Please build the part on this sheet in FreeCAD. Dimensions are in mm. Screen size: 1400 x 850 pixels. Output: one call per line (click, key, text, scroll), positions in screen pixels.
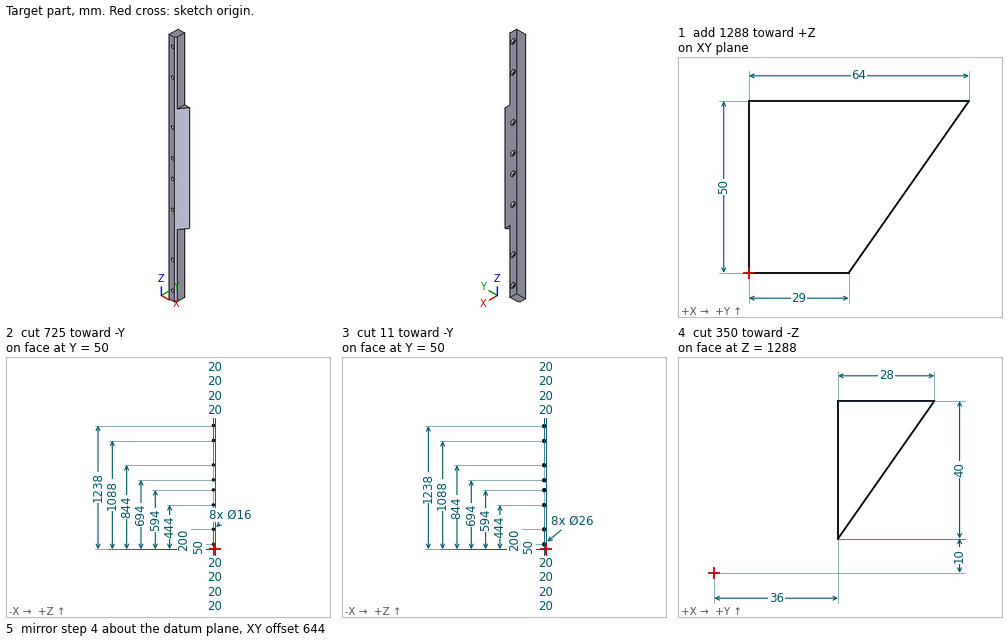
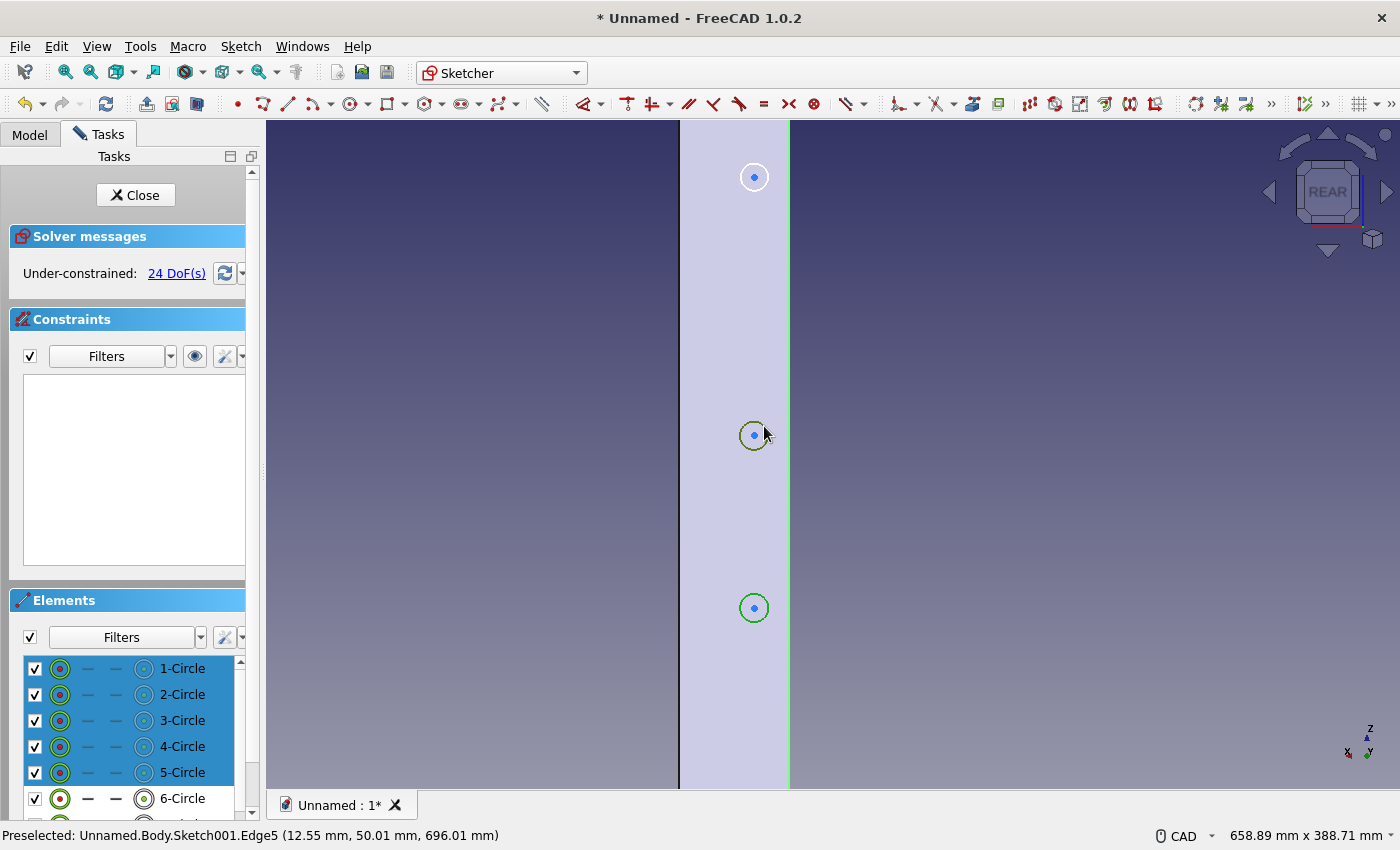
click(764, 167)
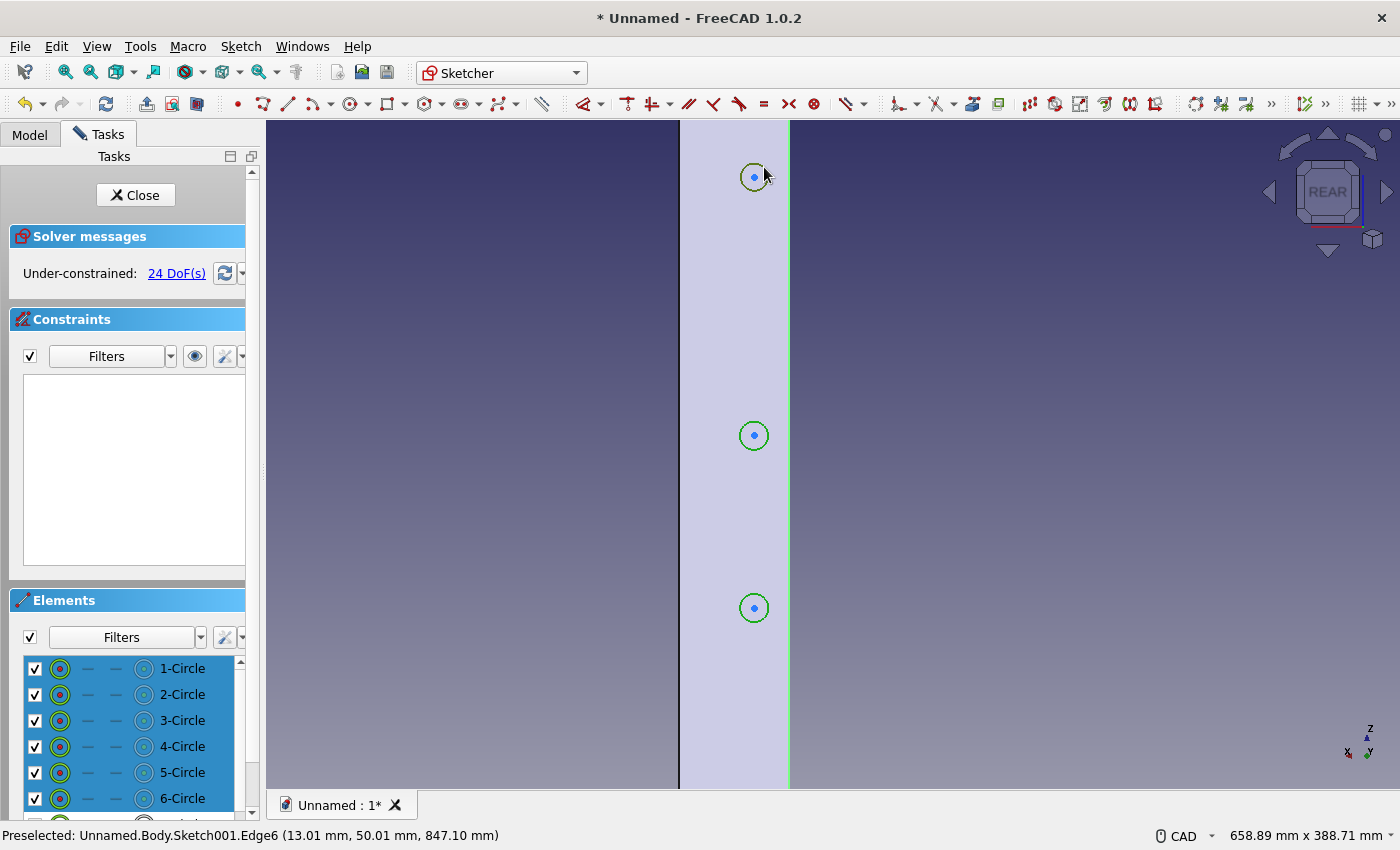
scroll(764, 429, down, 8)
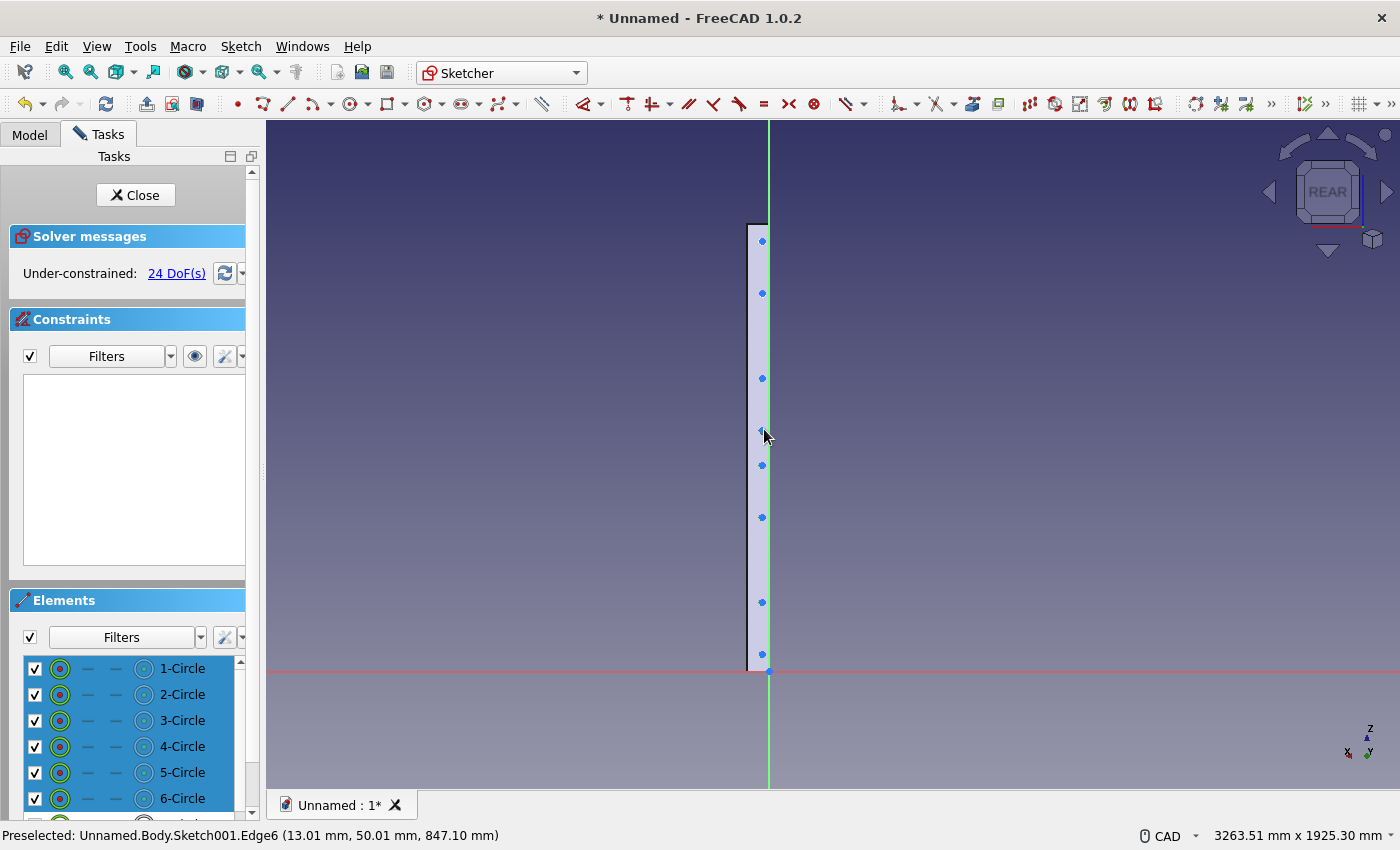
scroll(765, 292, up, 8)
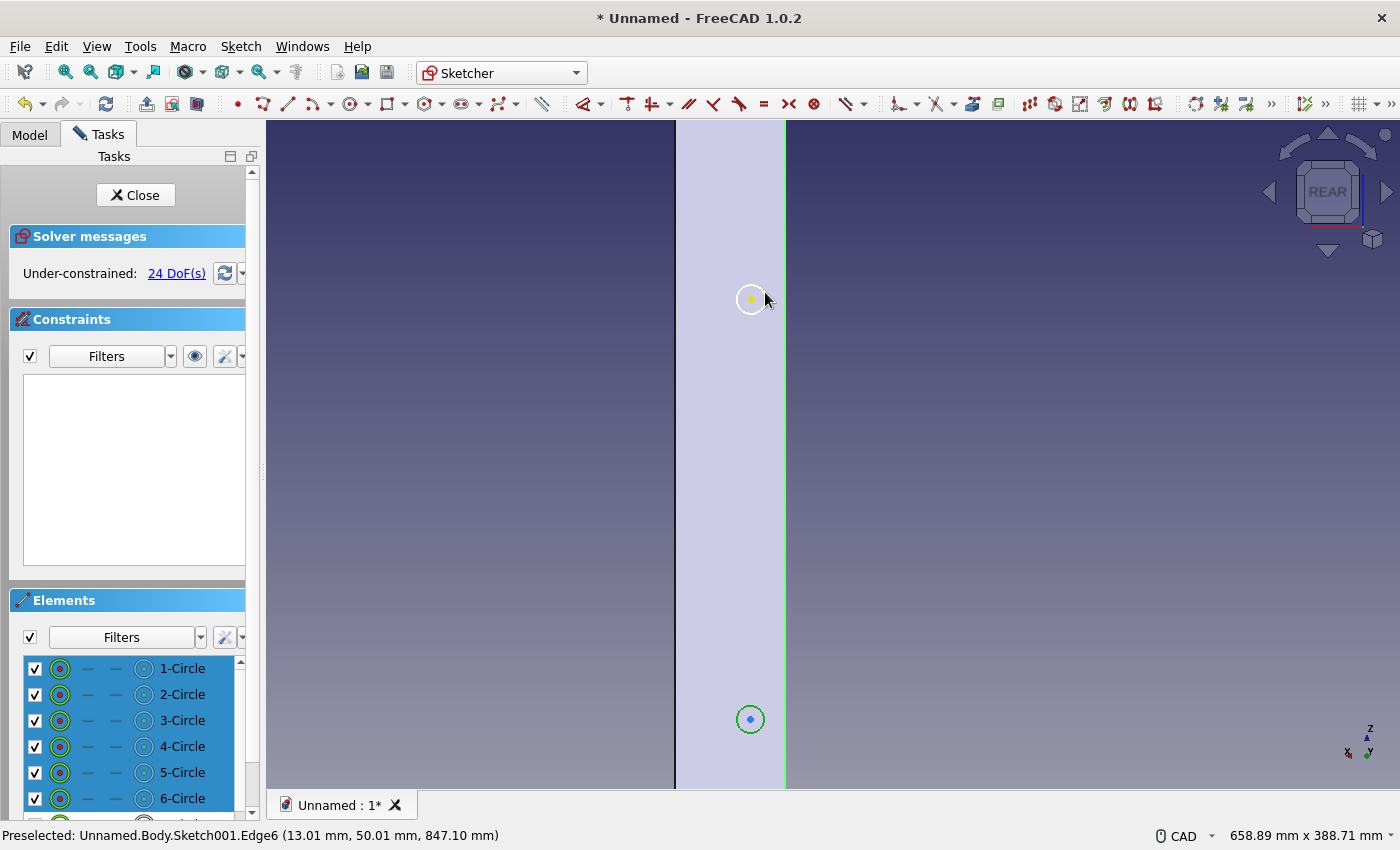
click(761, 289)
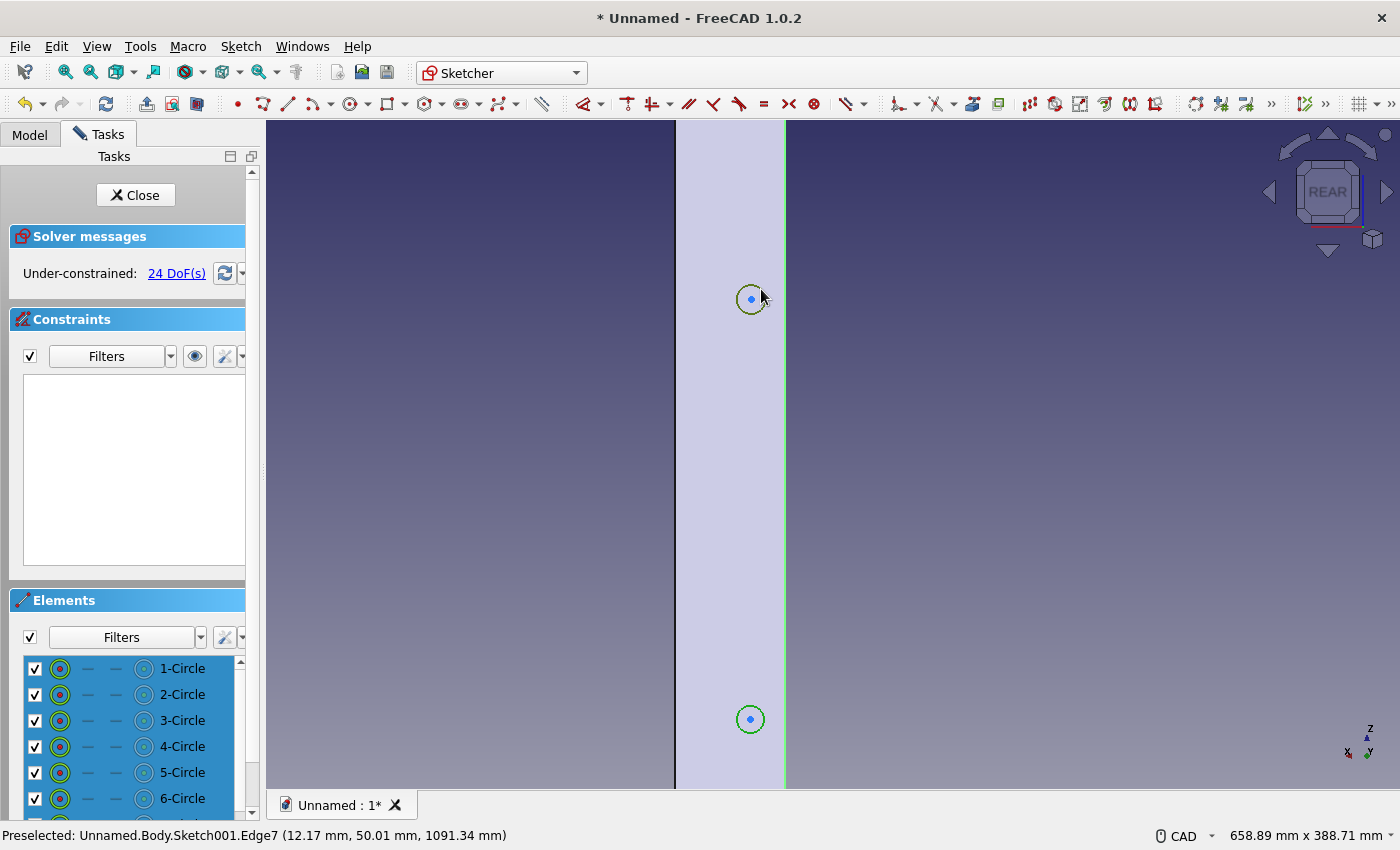
scroll(765, 292, down, 8)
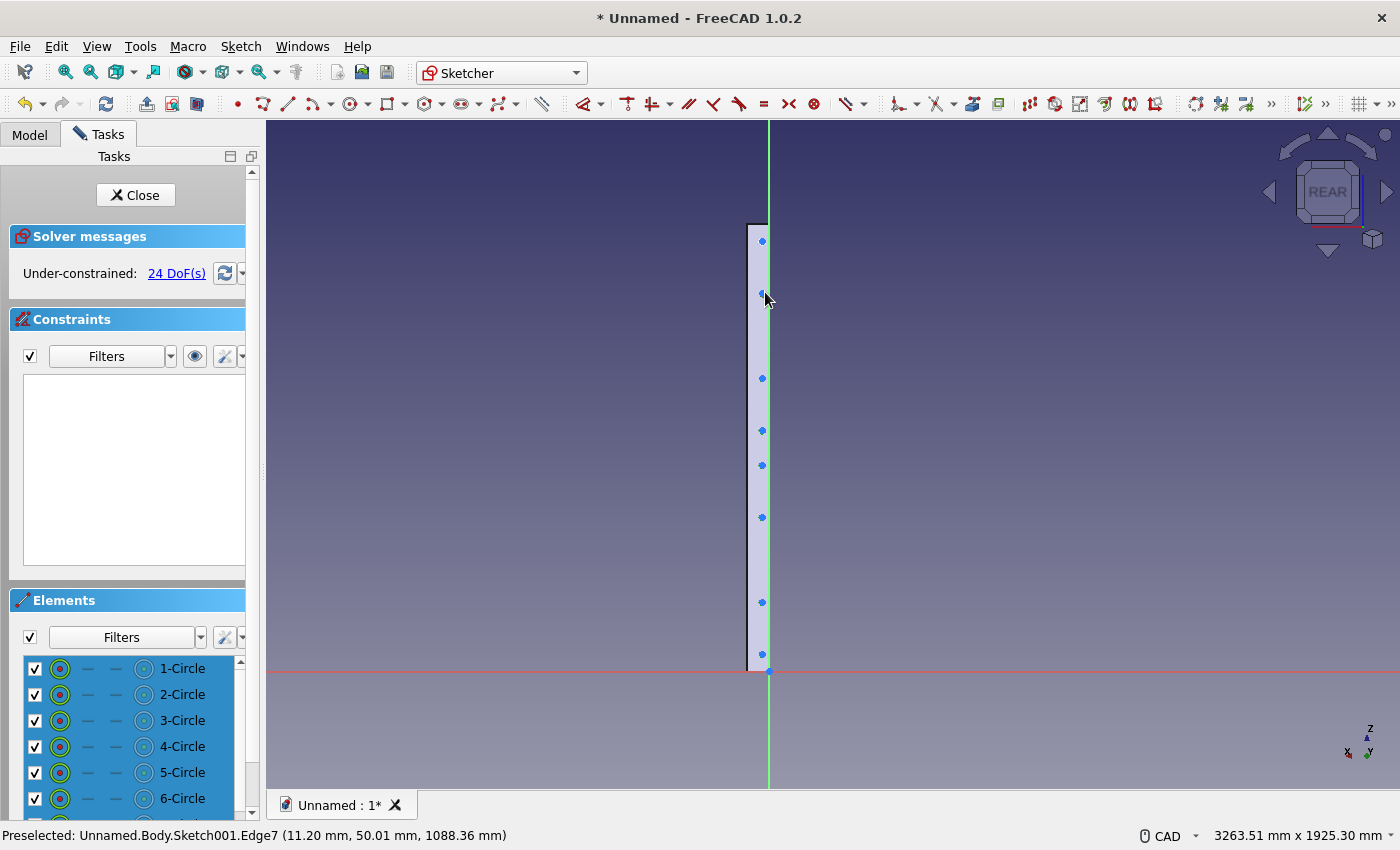
scroll(764, 240, up, 8)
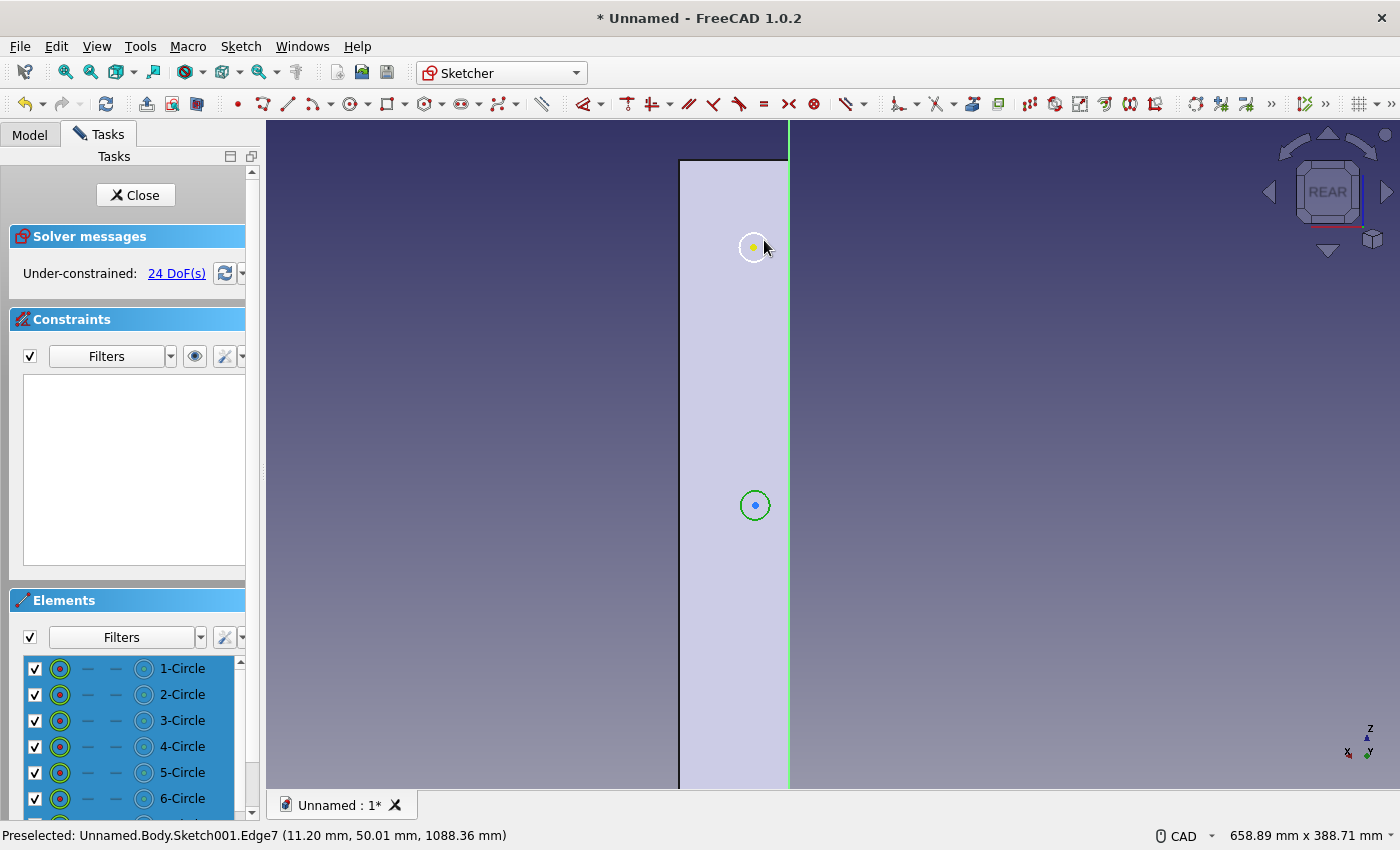
click(764, 237)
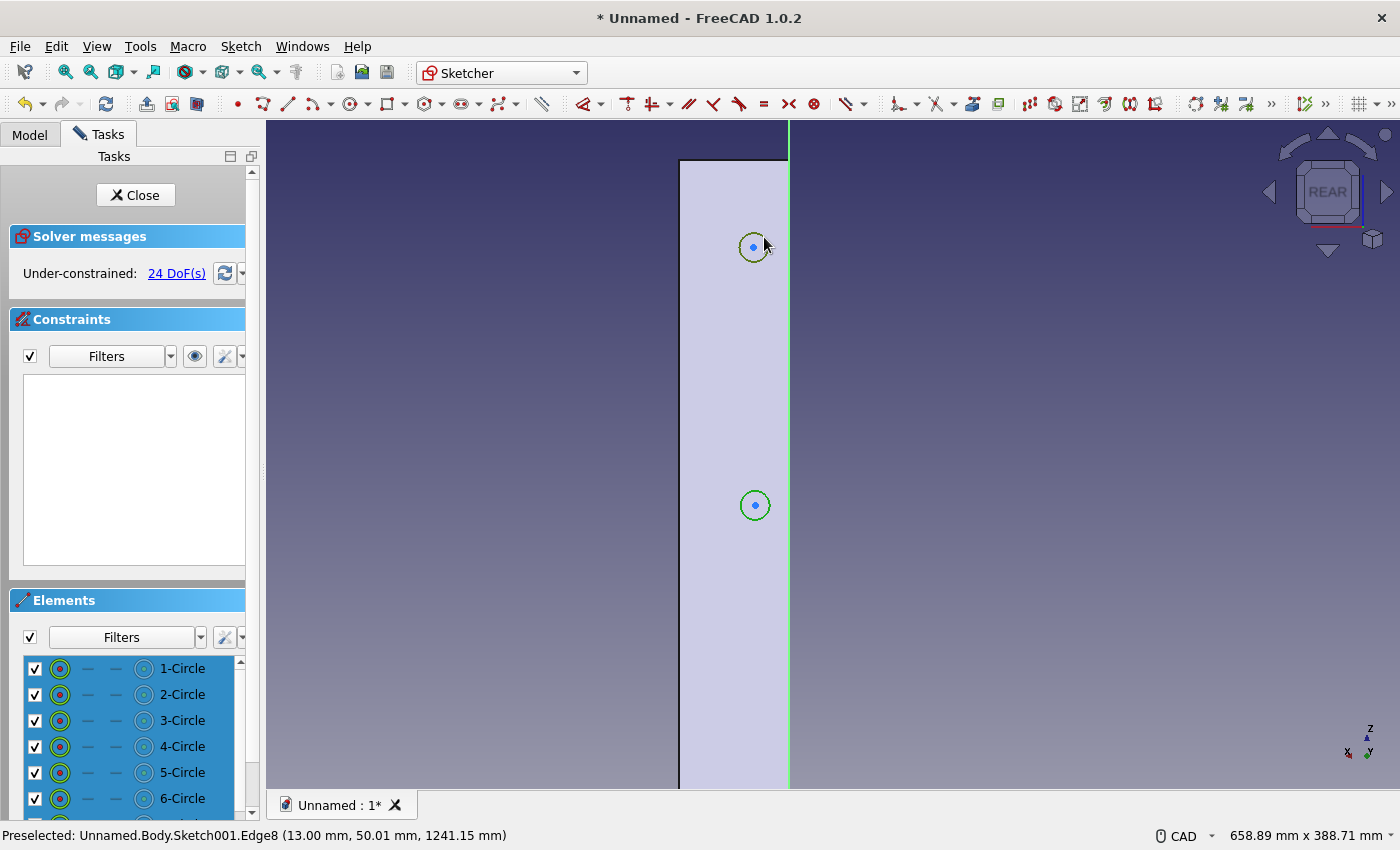
click(764, 104)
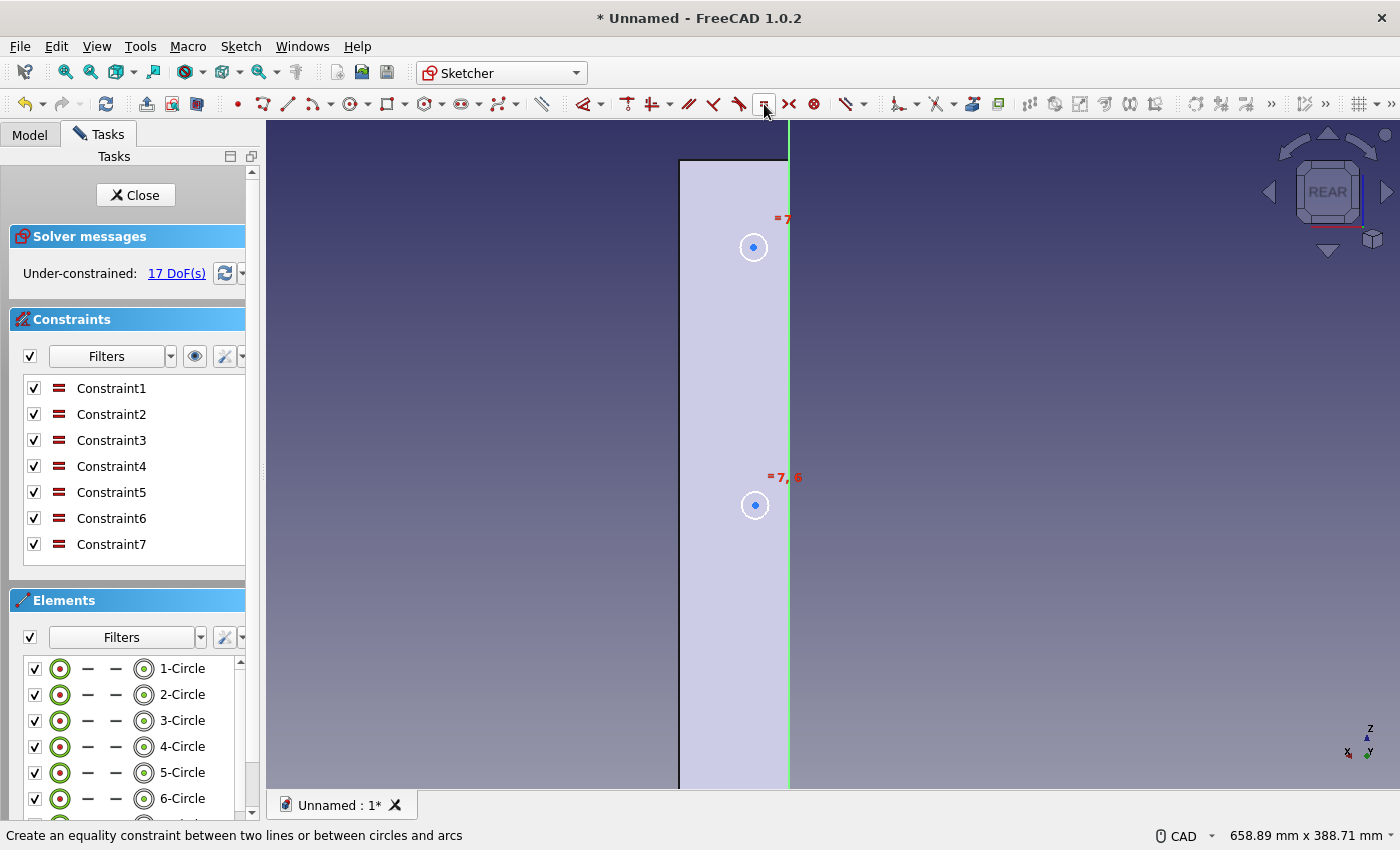
scroll(764, 239, down, 8)